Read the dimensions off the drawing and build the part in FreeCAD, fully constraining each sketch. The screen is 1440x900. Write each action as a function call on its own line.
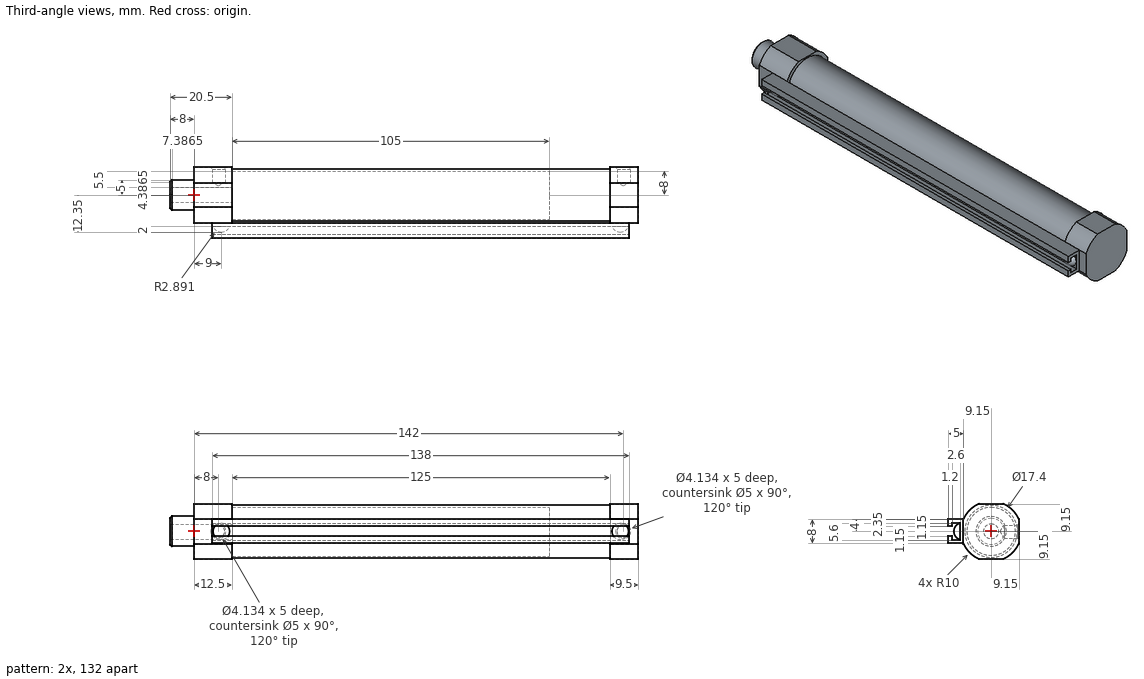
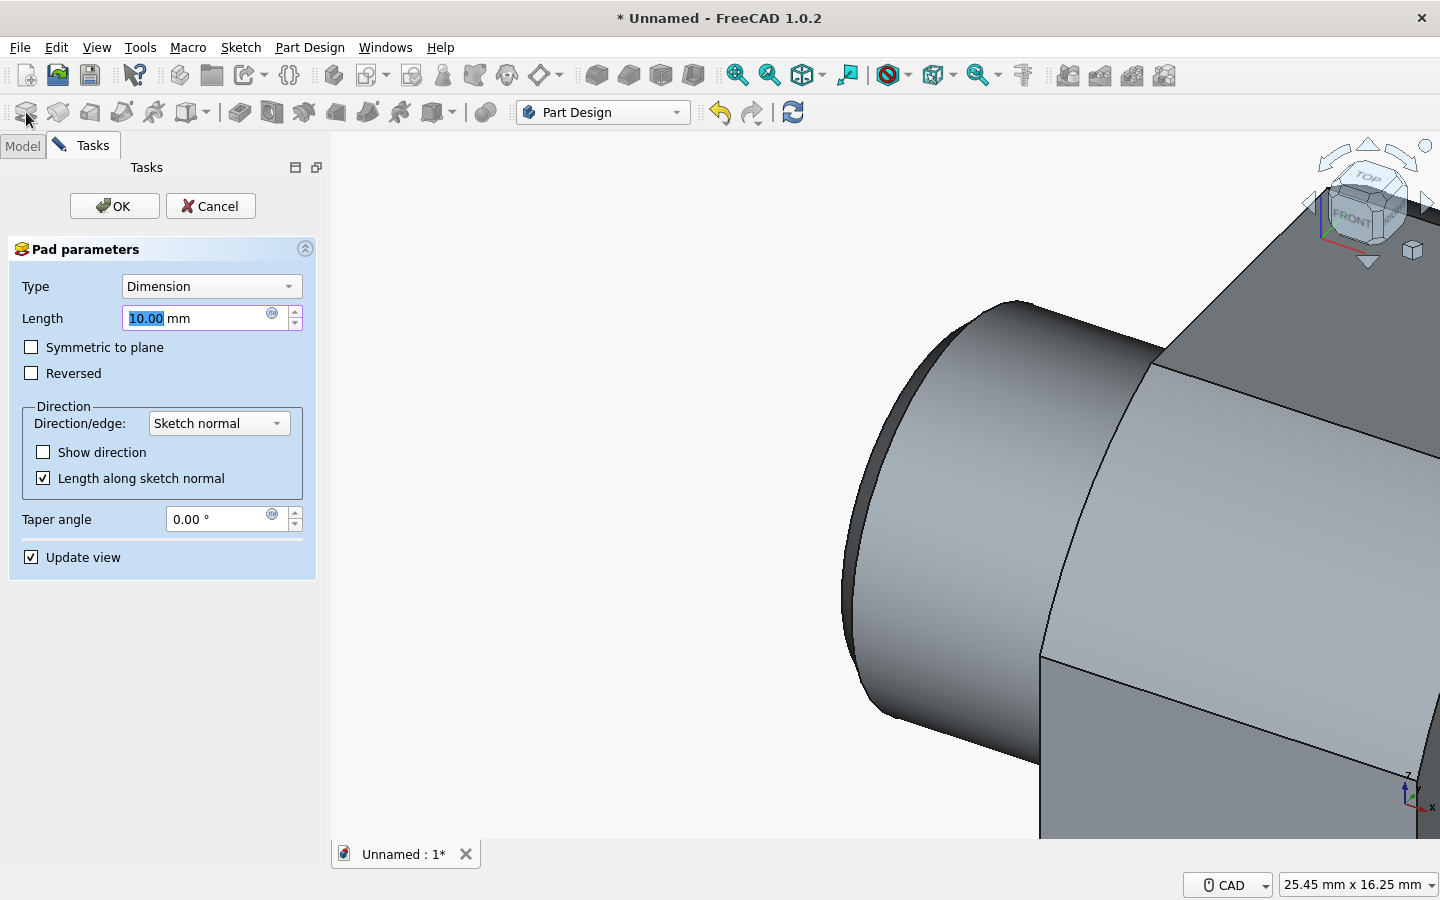
text(12.5)
key(Tab)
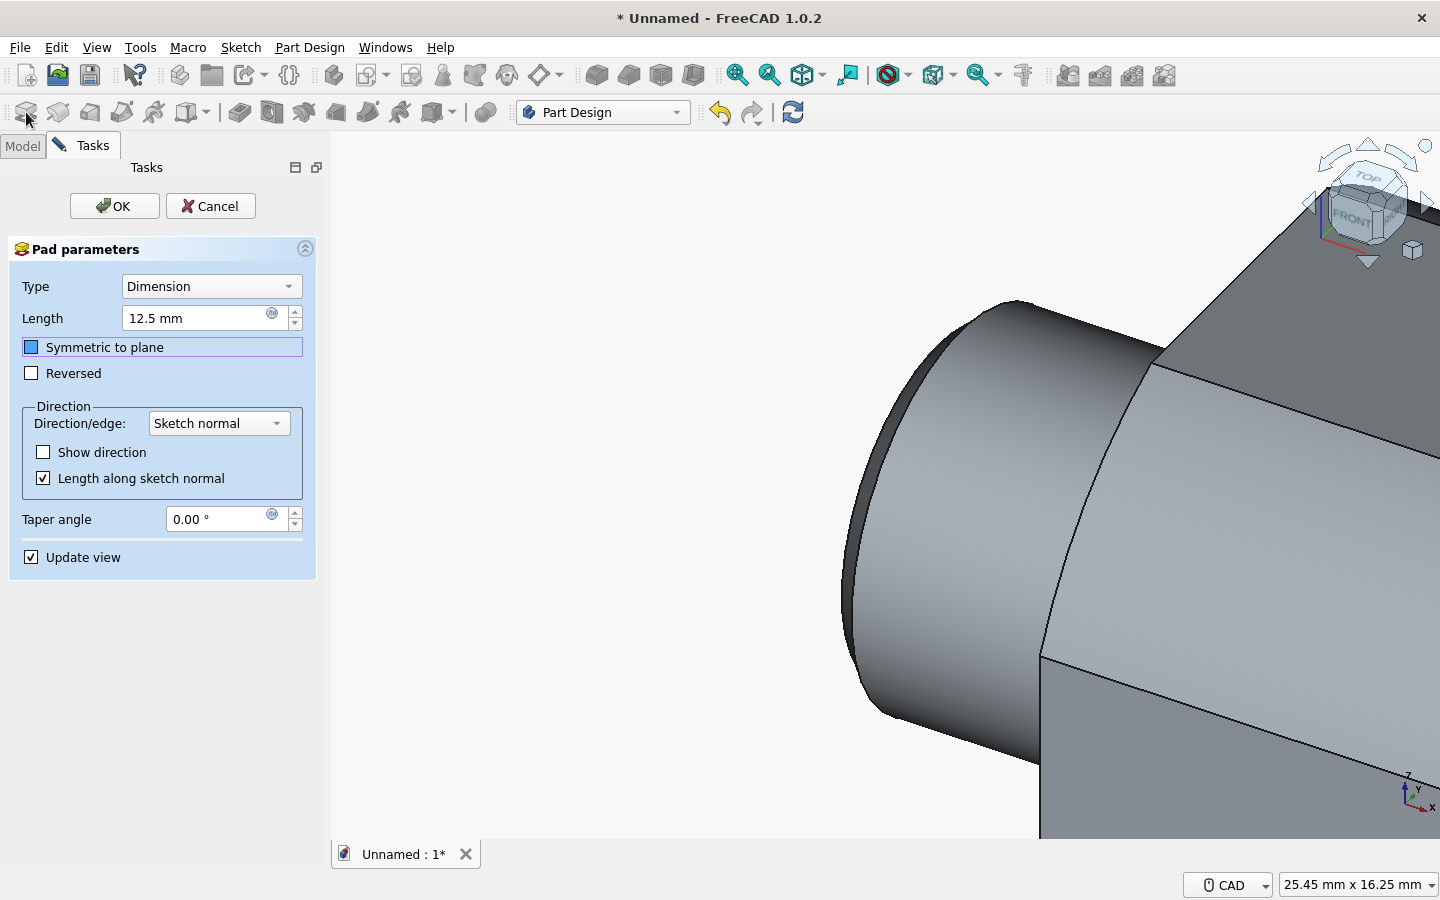
click(115, 206)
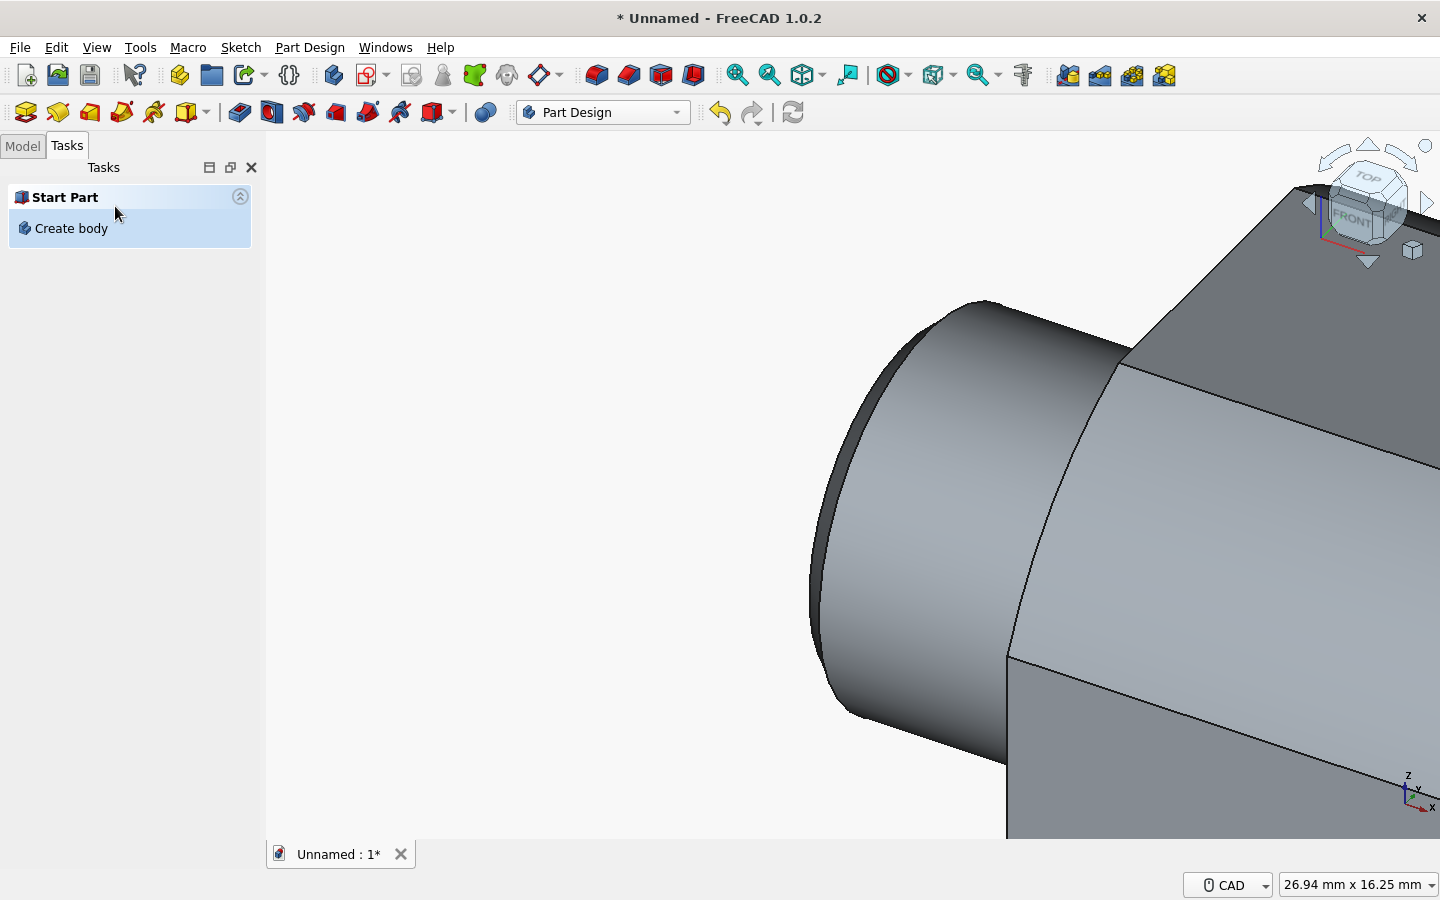
click(738, 76)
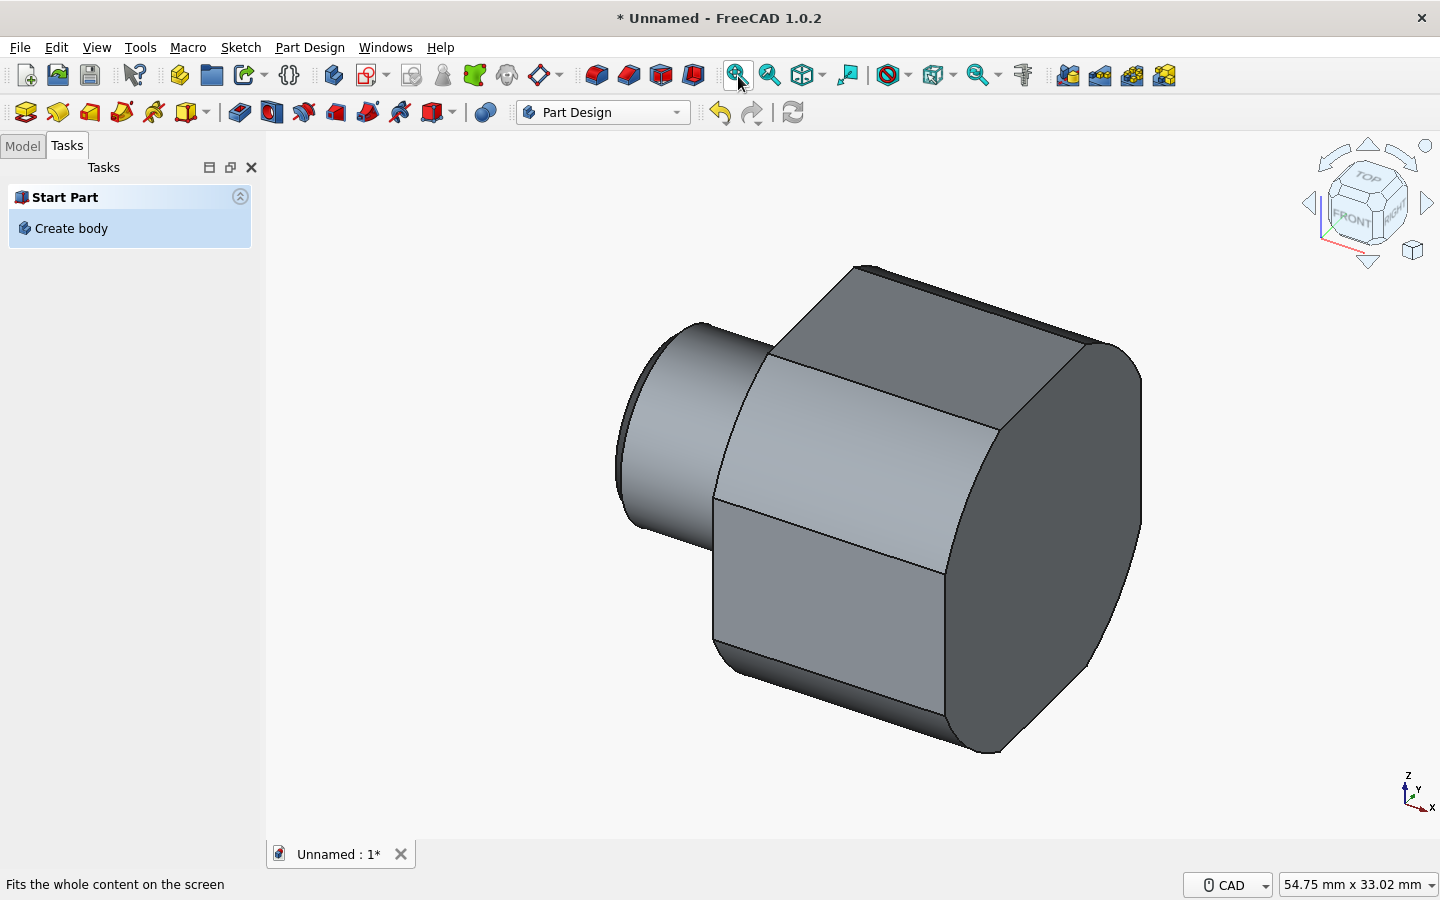
click(1043, 547)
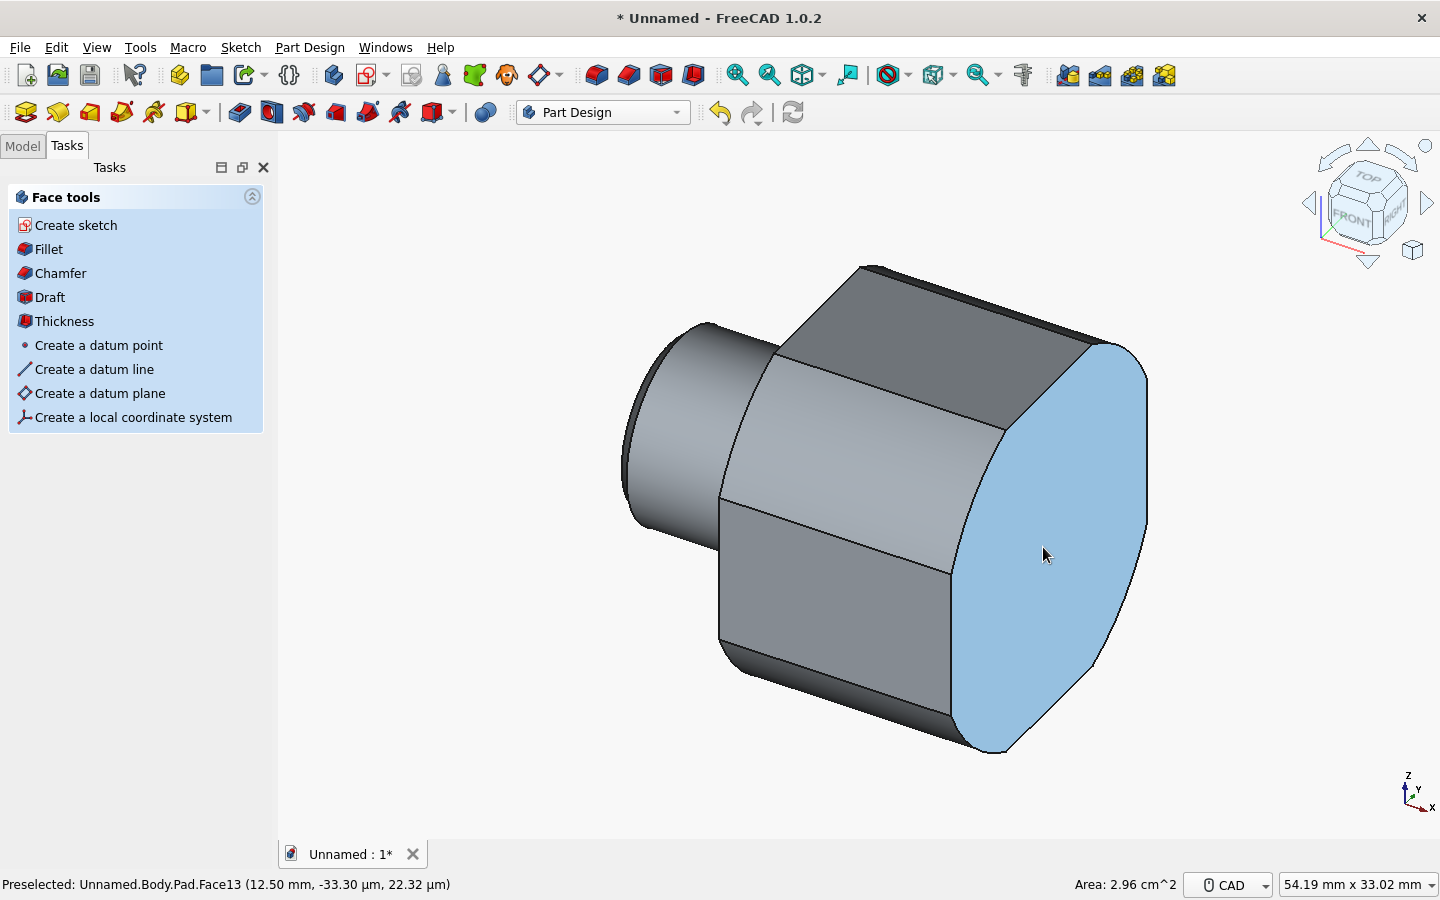
click(366, 76)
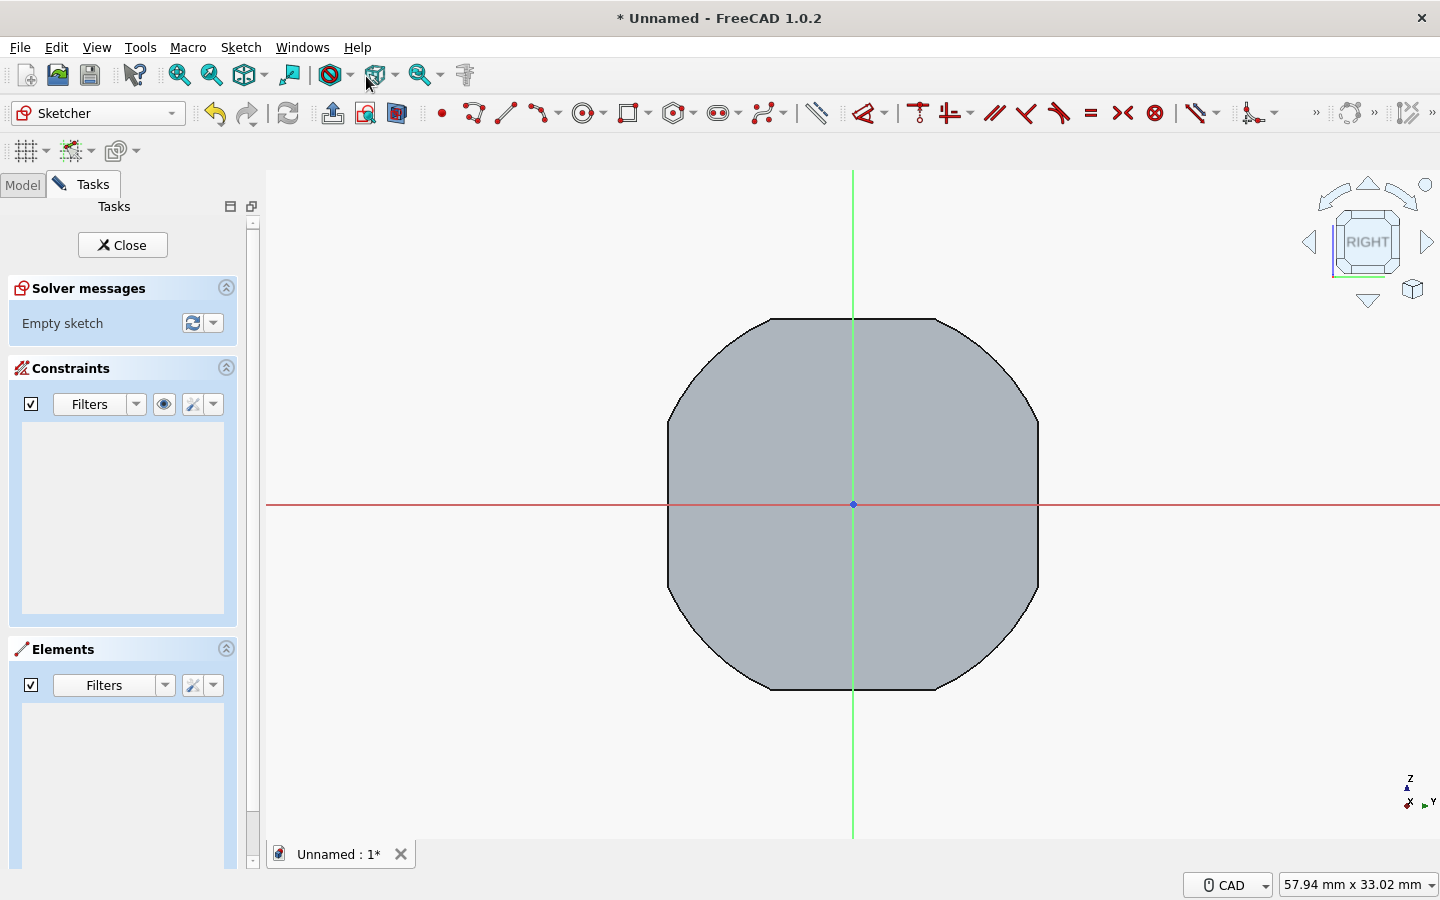
click(584, 114)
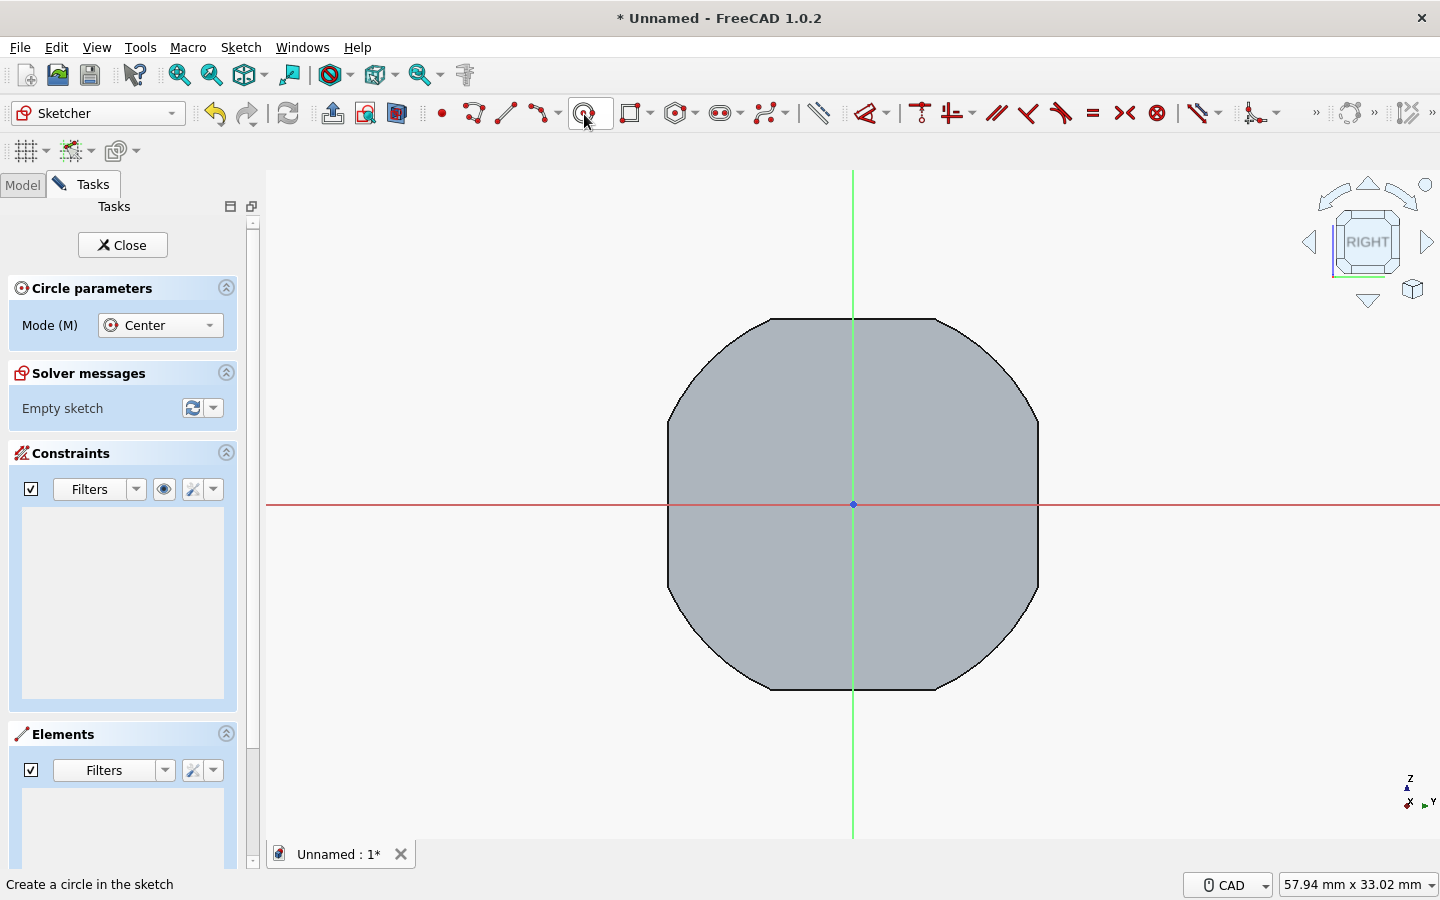
click(853, 504)
click(978, 380)
key(Escape)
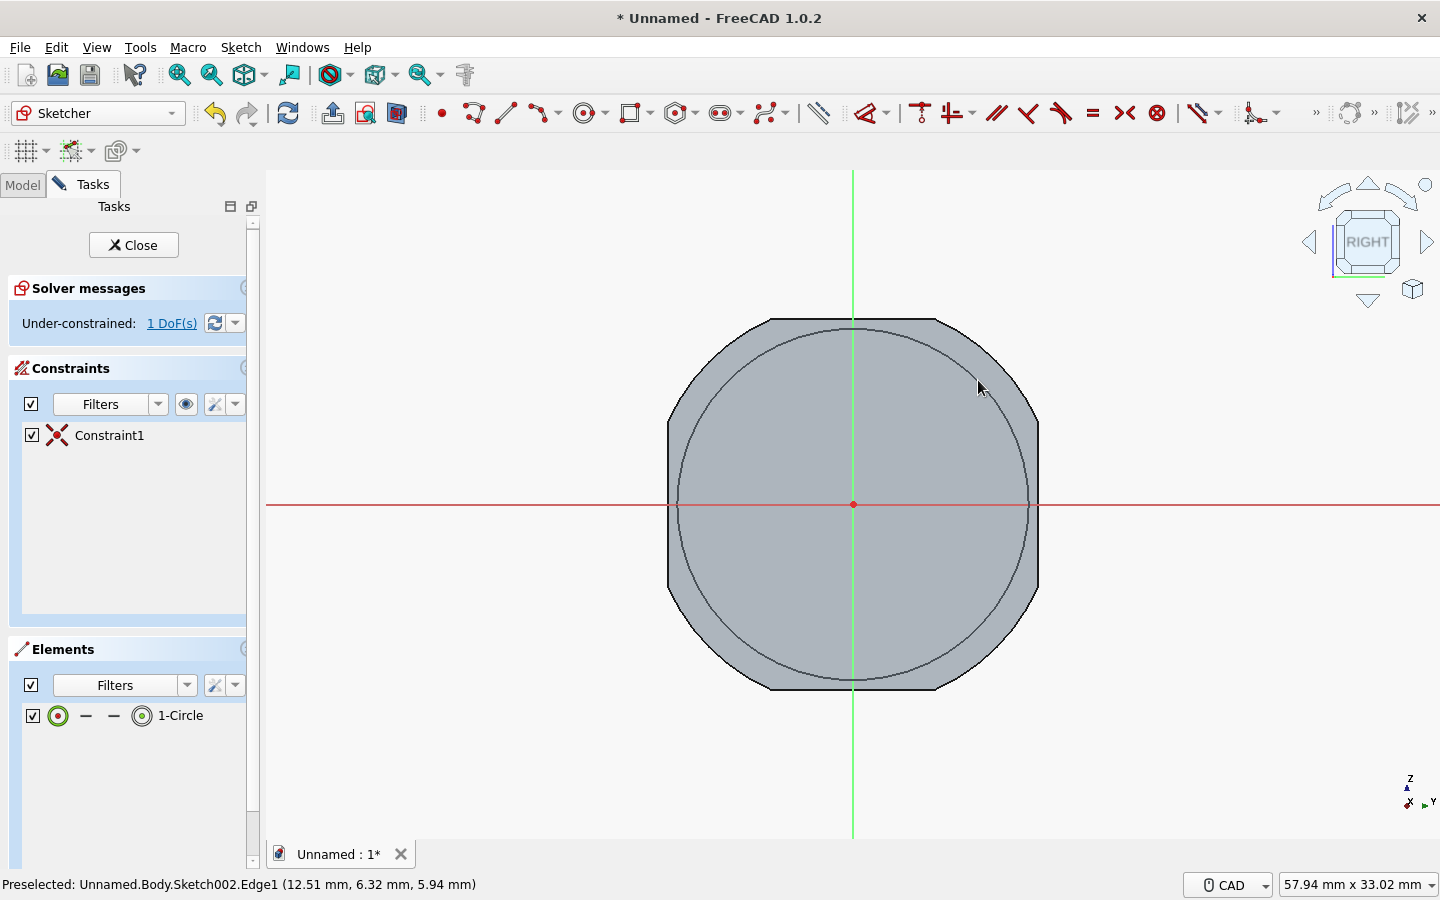
click(866, 114)